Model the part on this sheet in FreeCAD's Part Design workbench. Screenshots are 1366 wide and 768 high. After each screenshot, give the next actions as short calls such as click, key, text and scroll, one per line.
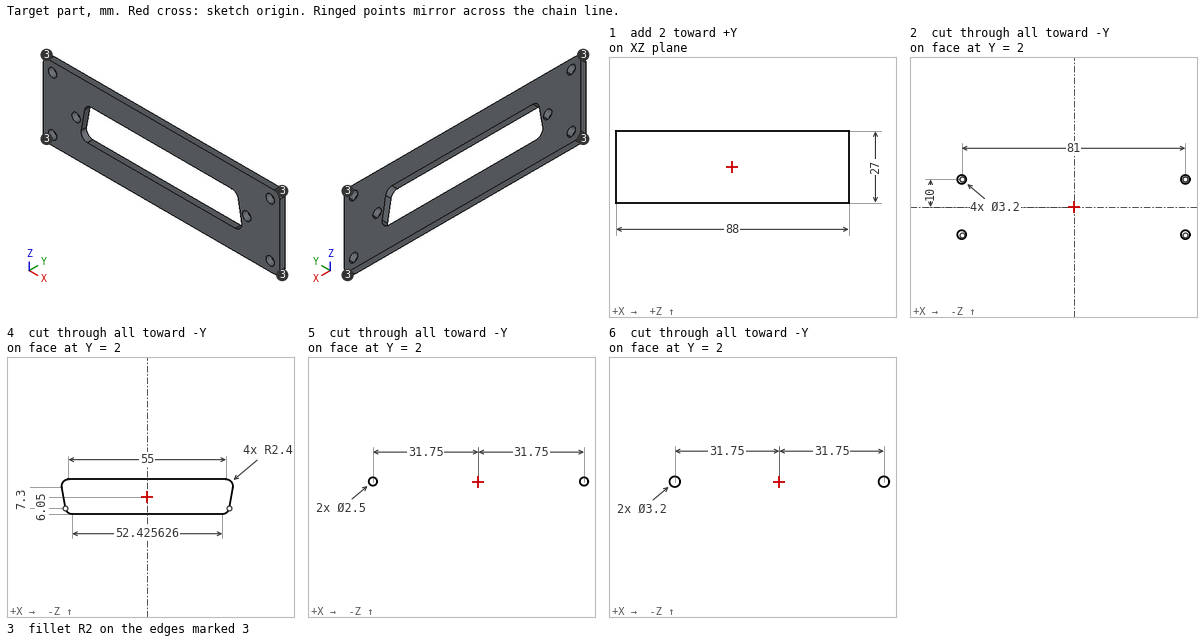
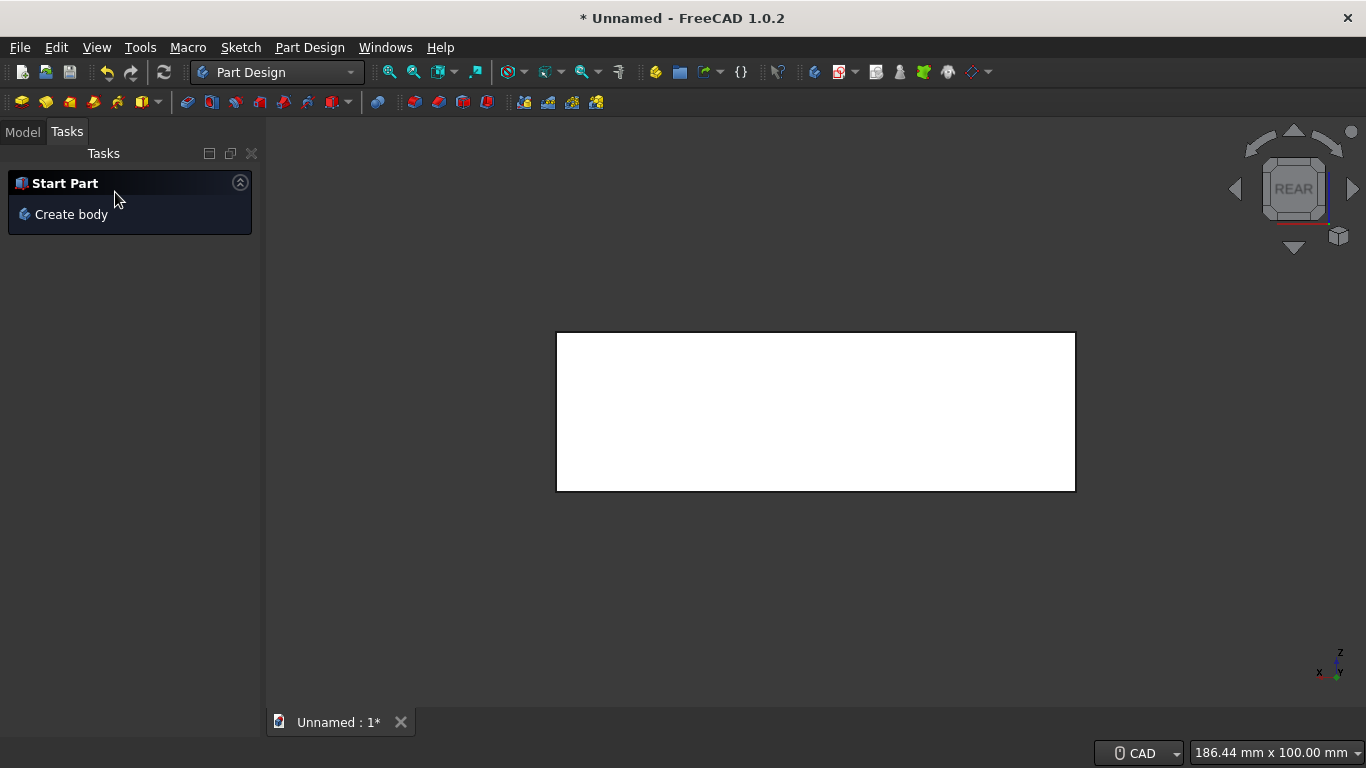
click(668, 411)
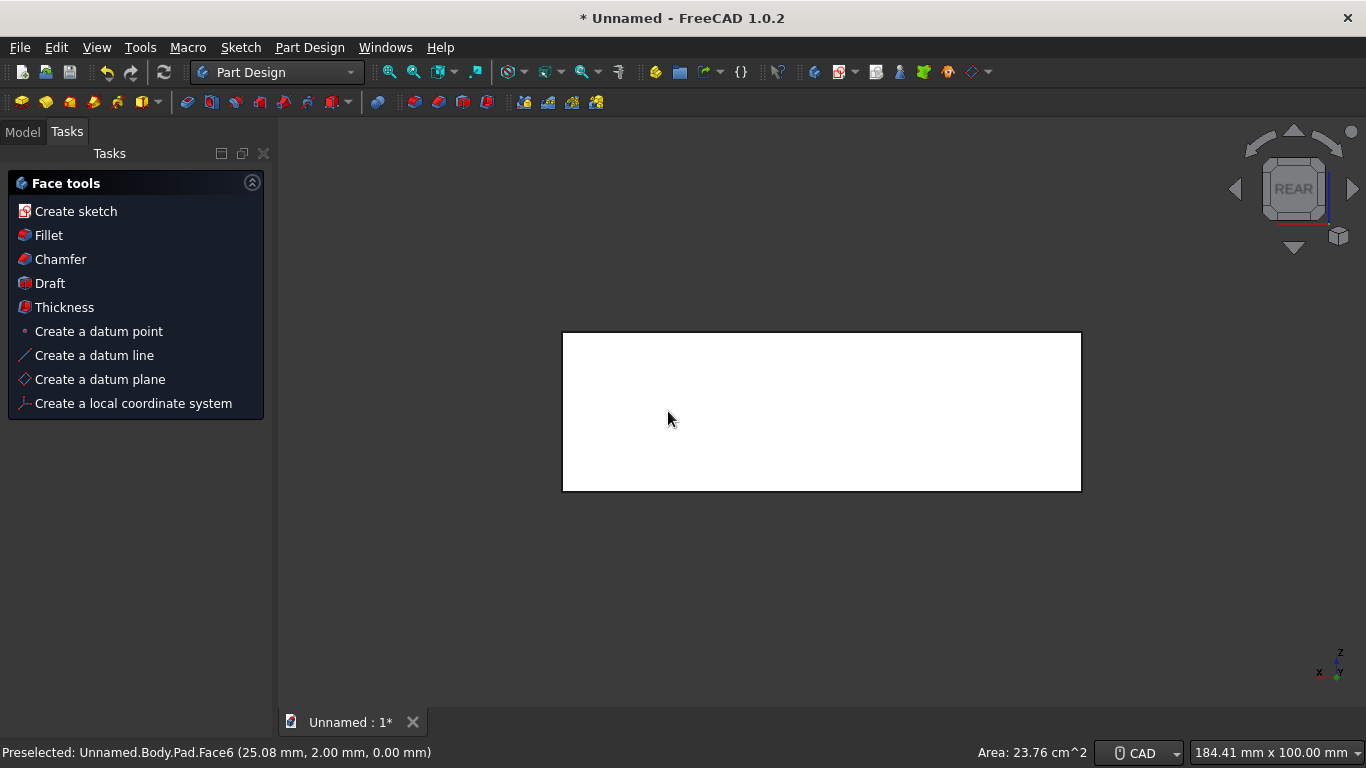
click(840, 72)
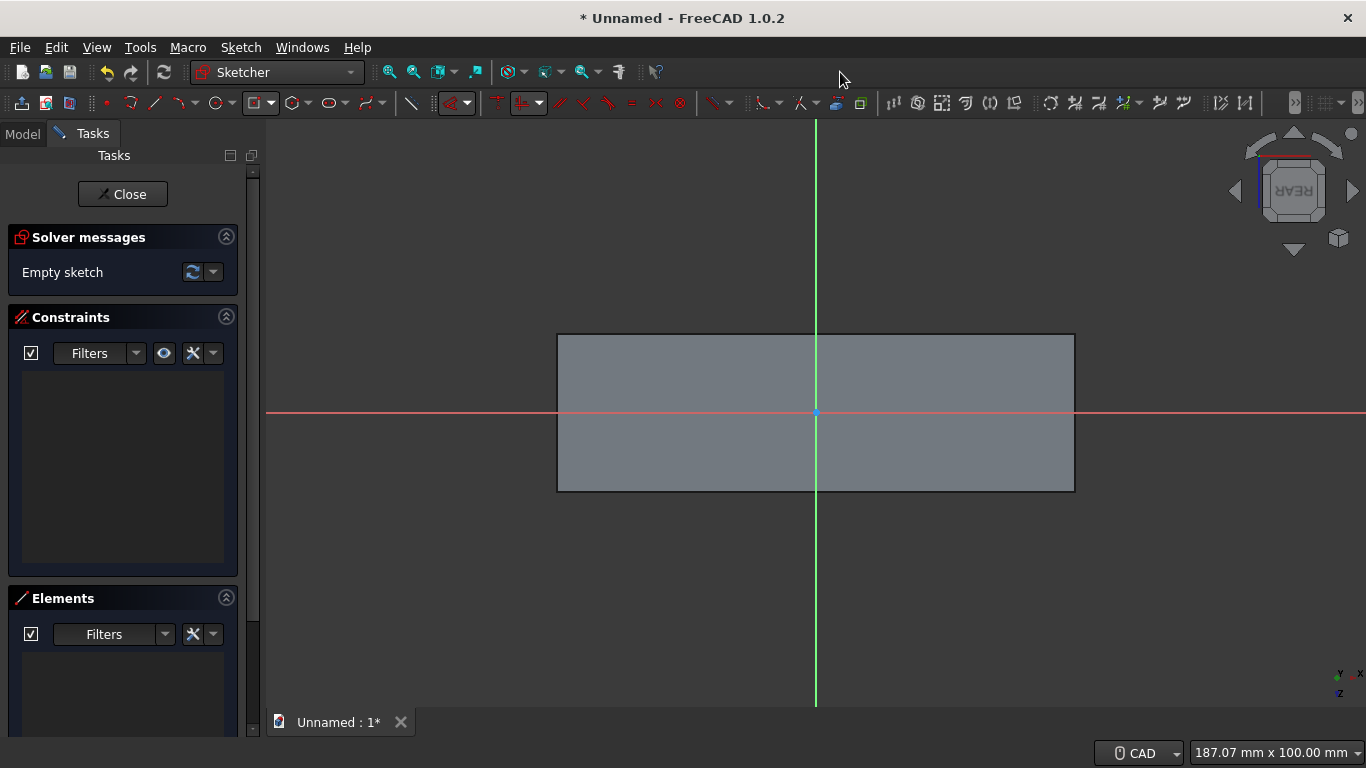
click(216, 104)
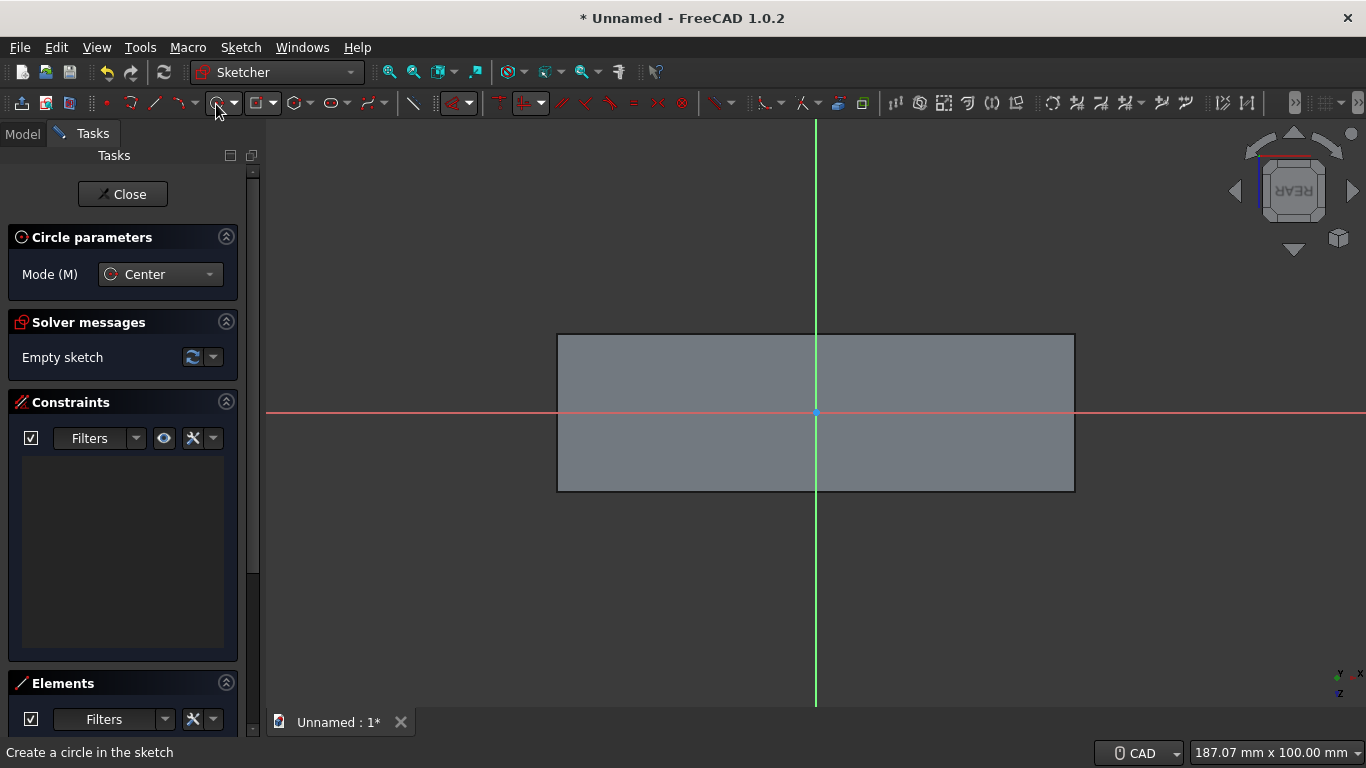
scroll(578, 354, up, 5)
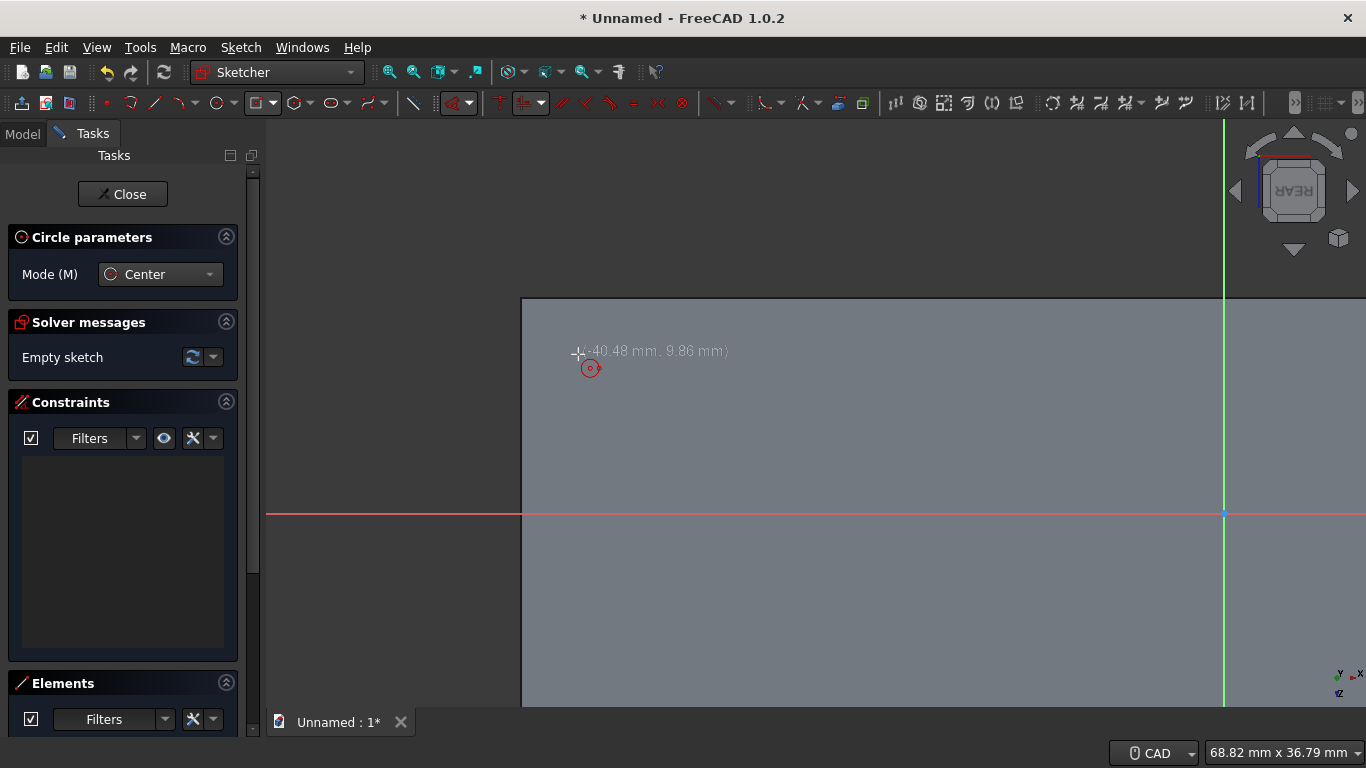
click(577, 354)
click(595, 336)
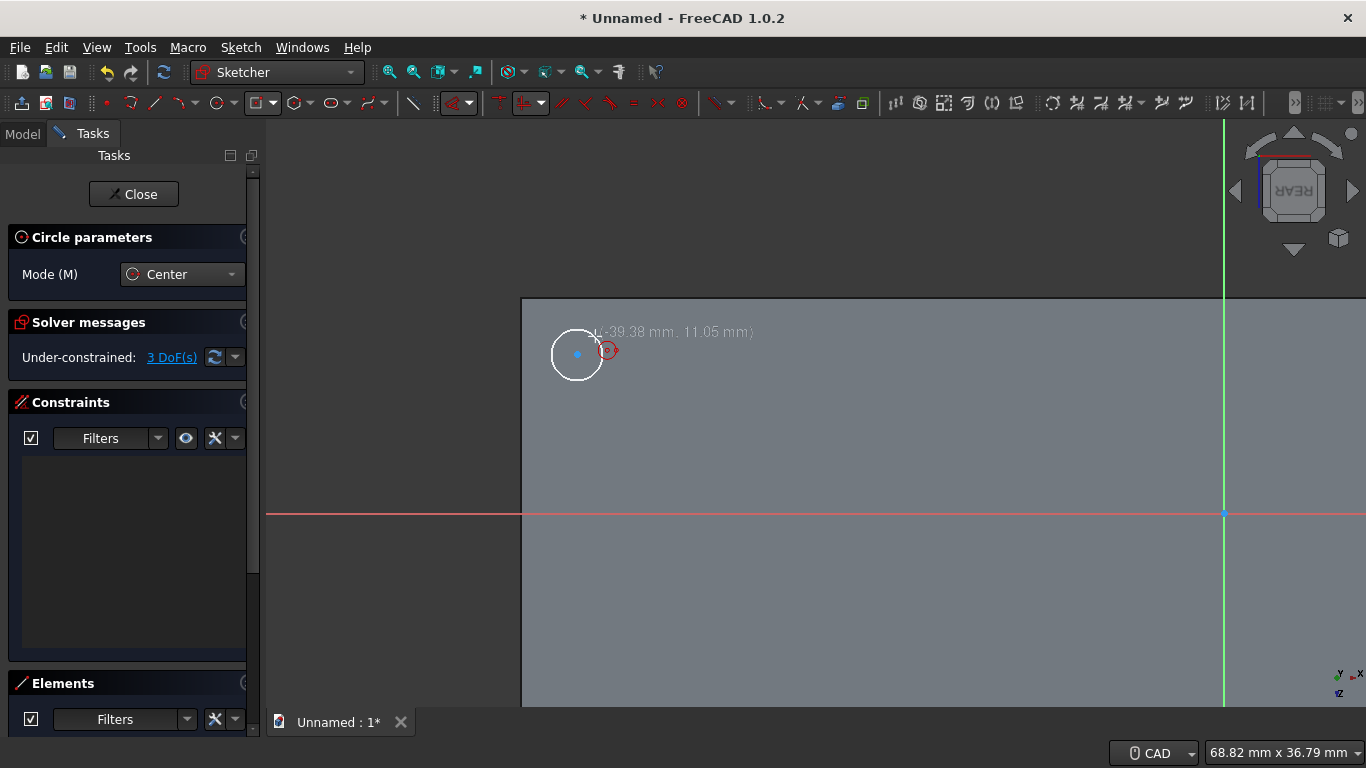
scroll(358, 331, down, 4)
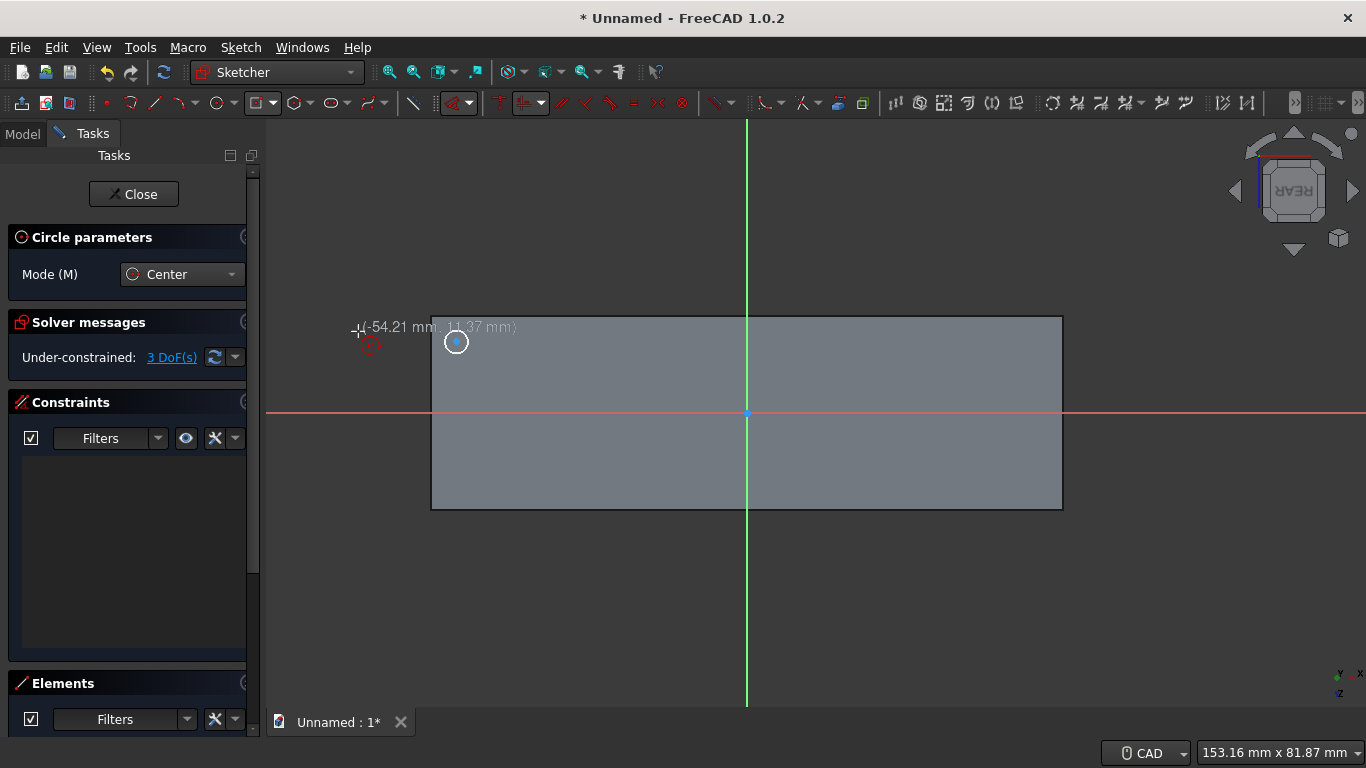
scroll(1038, 341, up, 4)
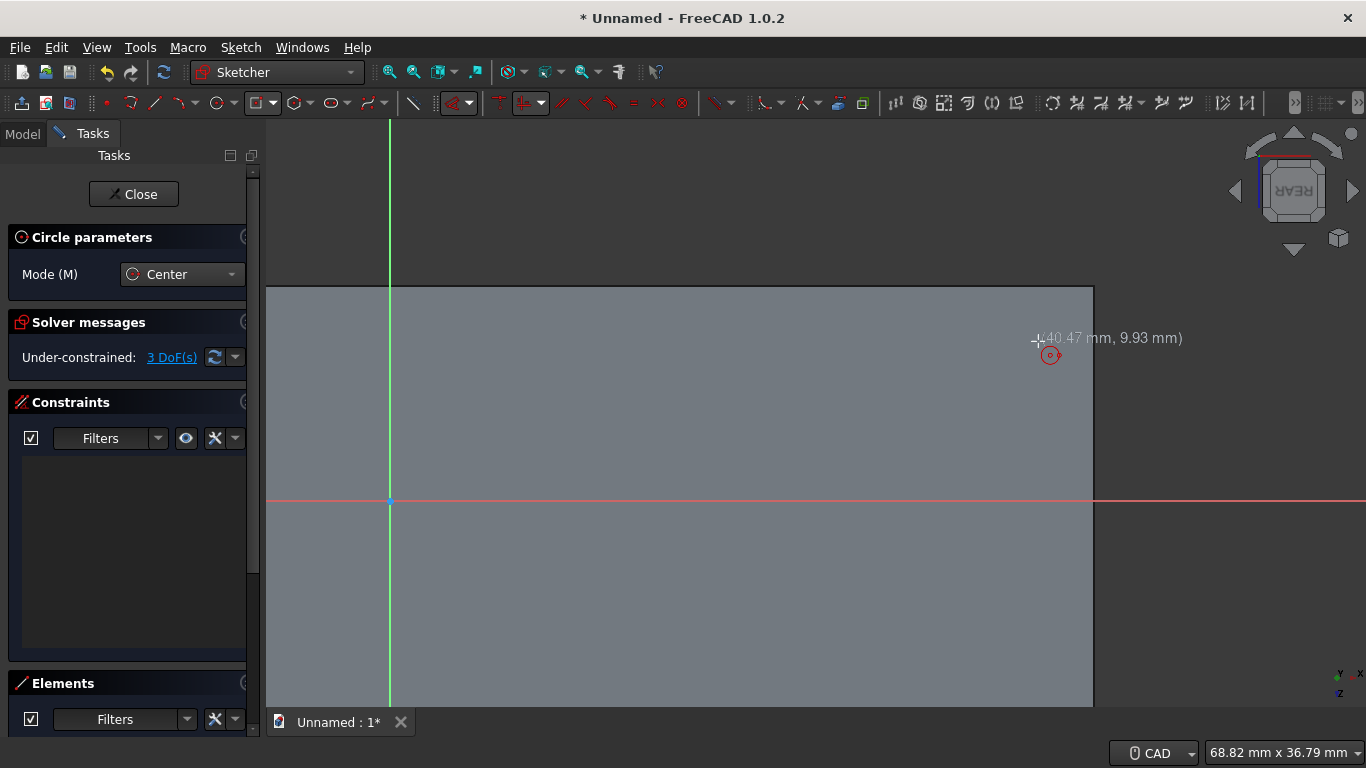
click(1038, 342)
click(1056, 323)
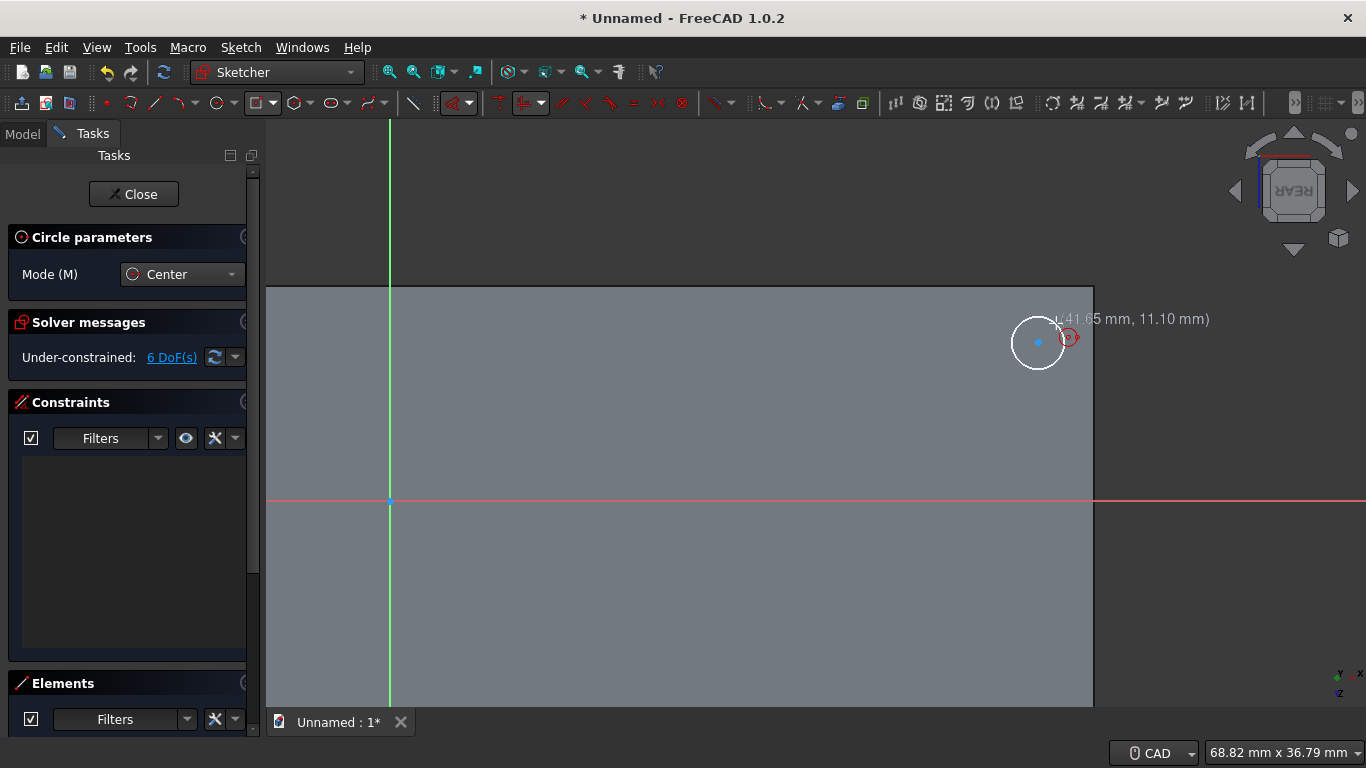
click(1038, 661)
click(1056, 643)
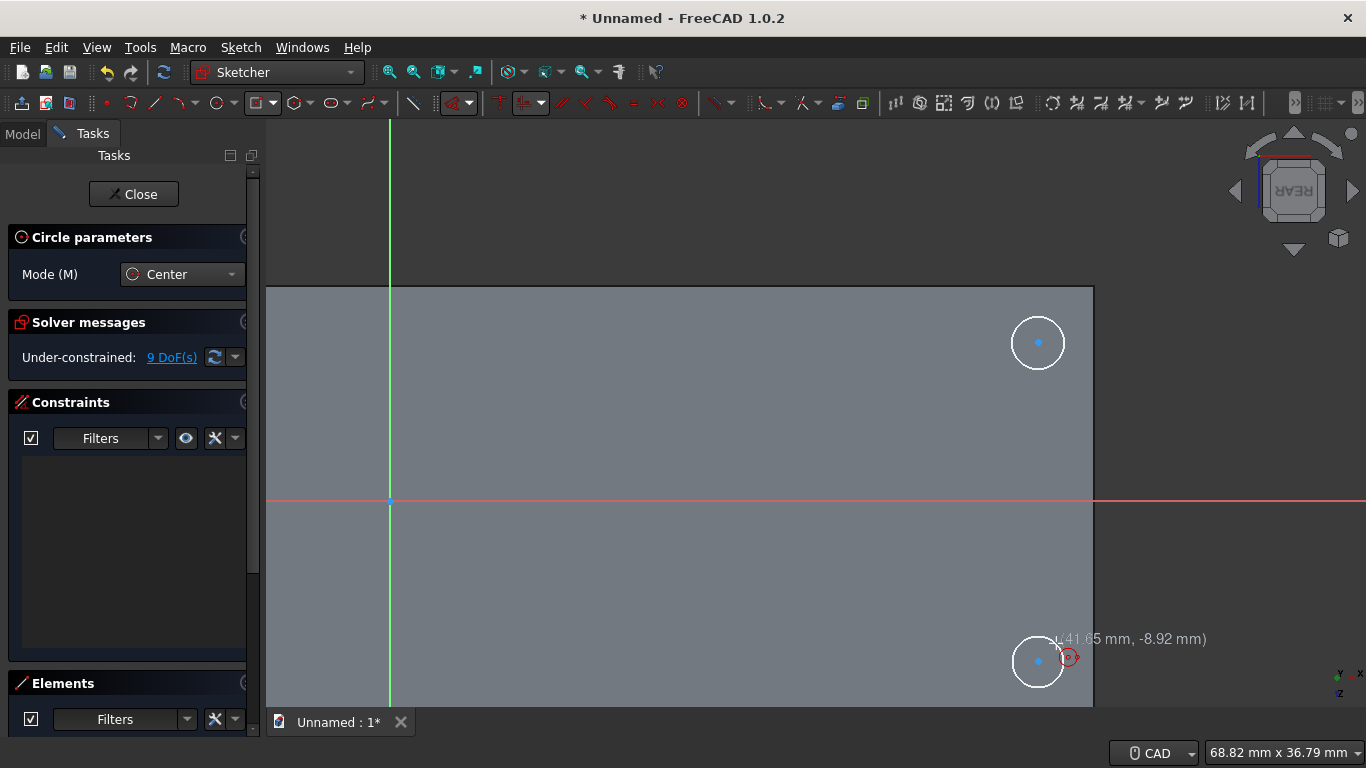
scroll(1039, 341, down, 4)